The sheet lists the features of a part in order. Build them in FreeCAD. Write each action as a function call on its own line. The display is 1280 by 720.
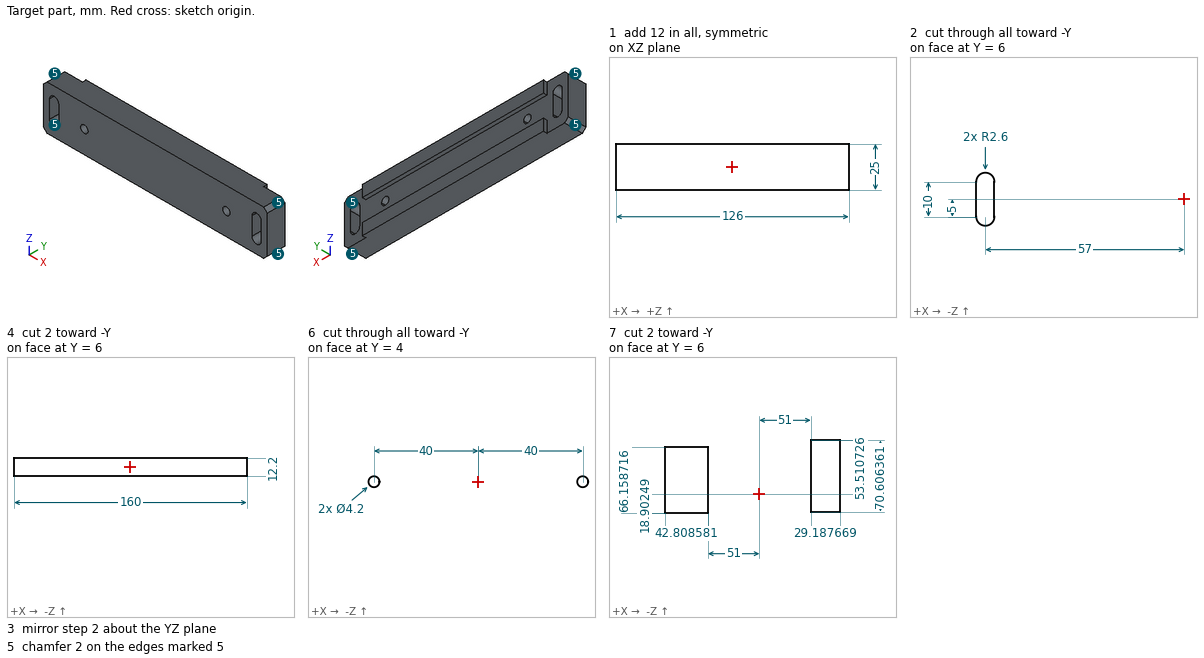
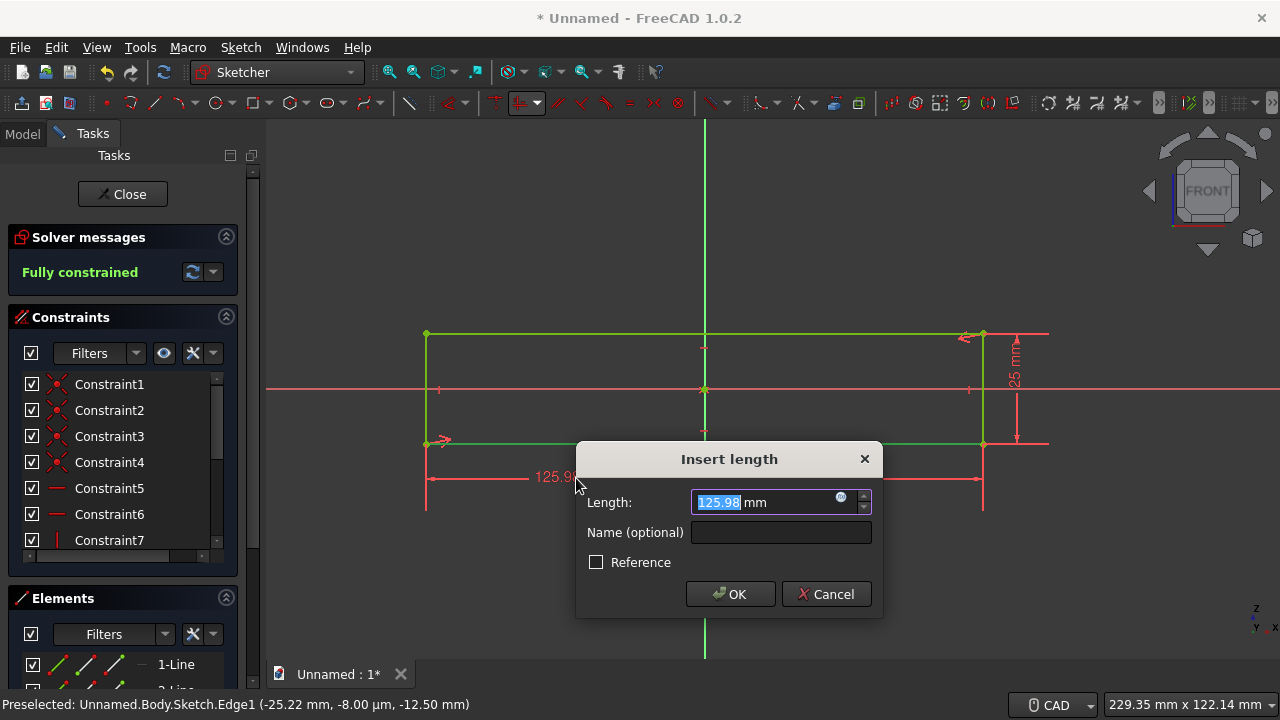
text(126)
key(Return)
key(Escape)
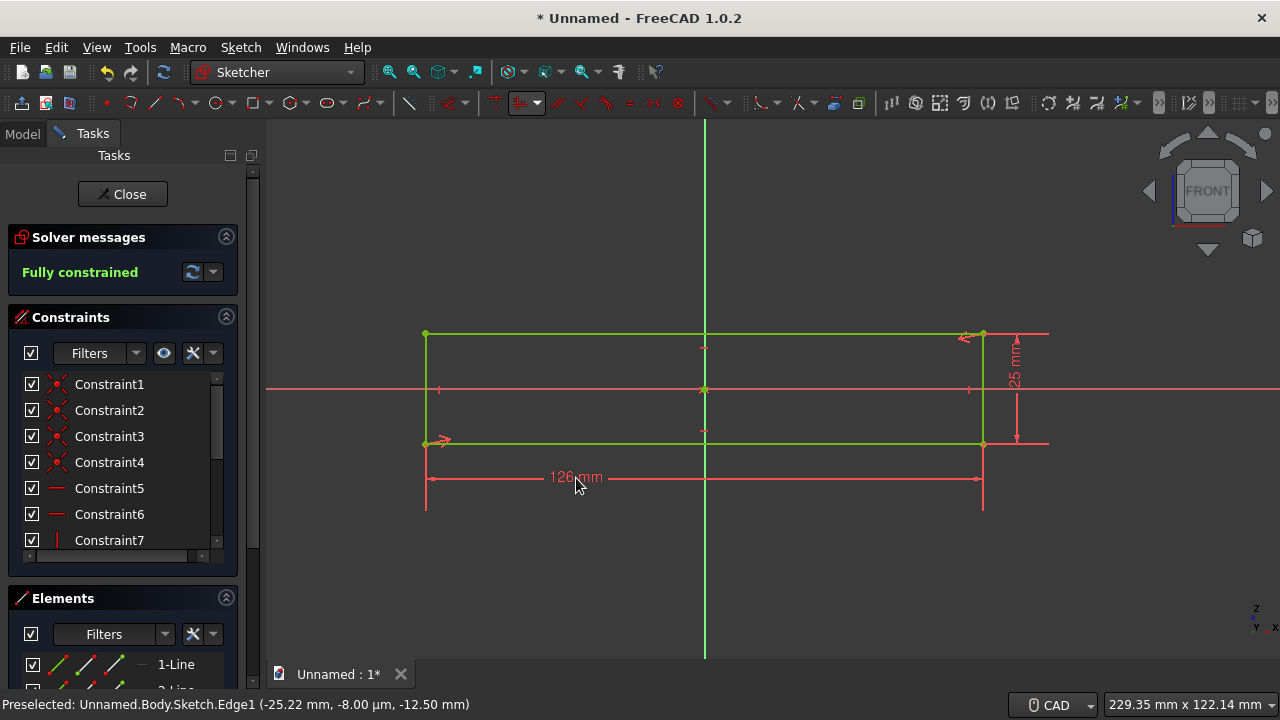
click(123, 194)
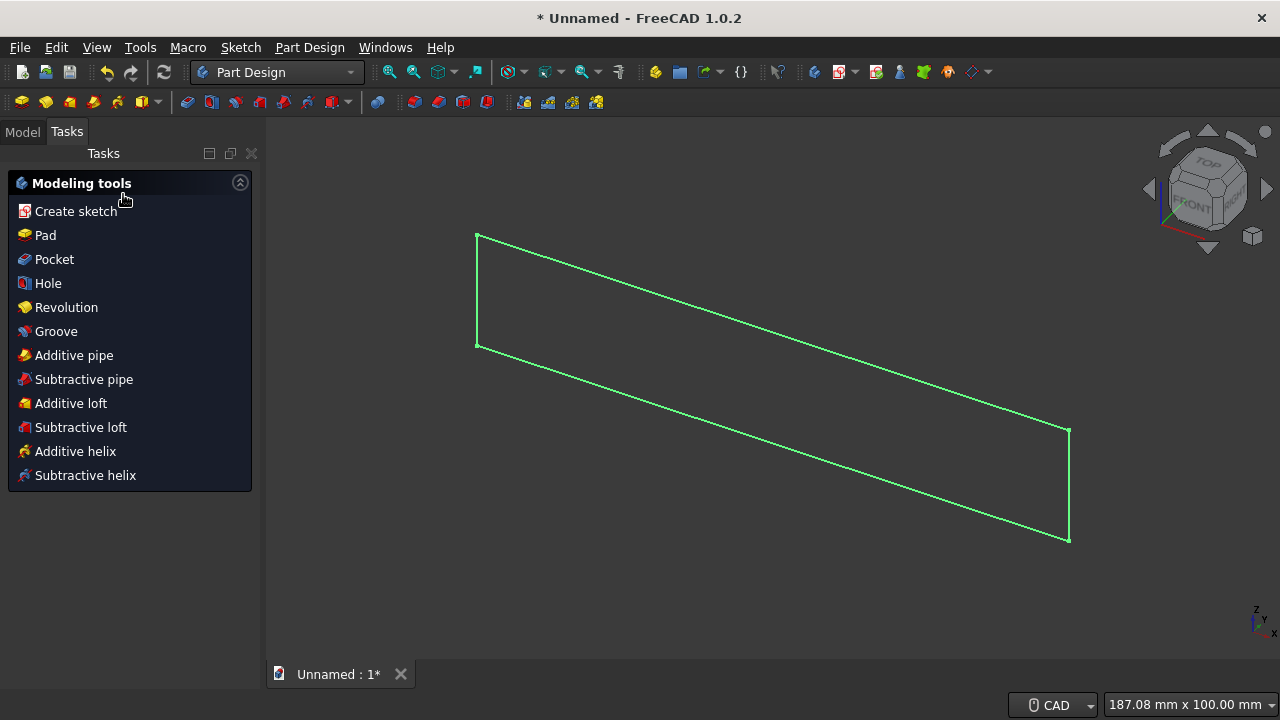
click(22, 102)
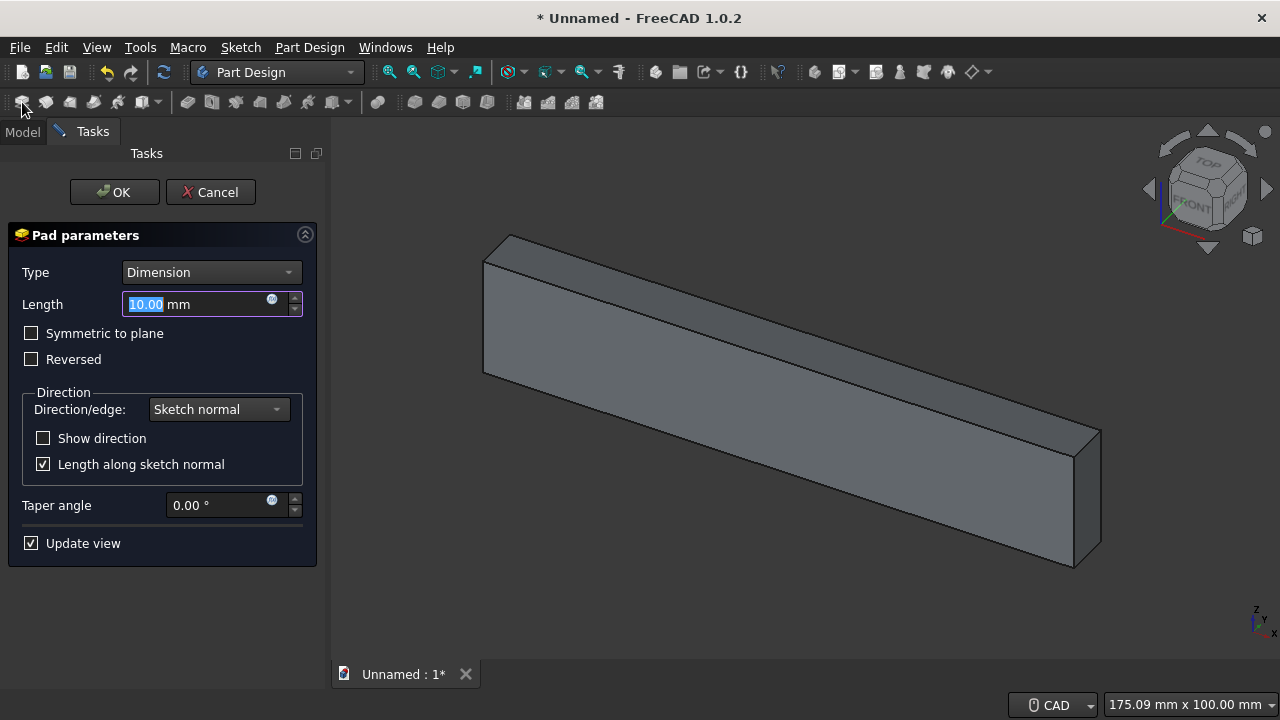
text(12)
key(Tab)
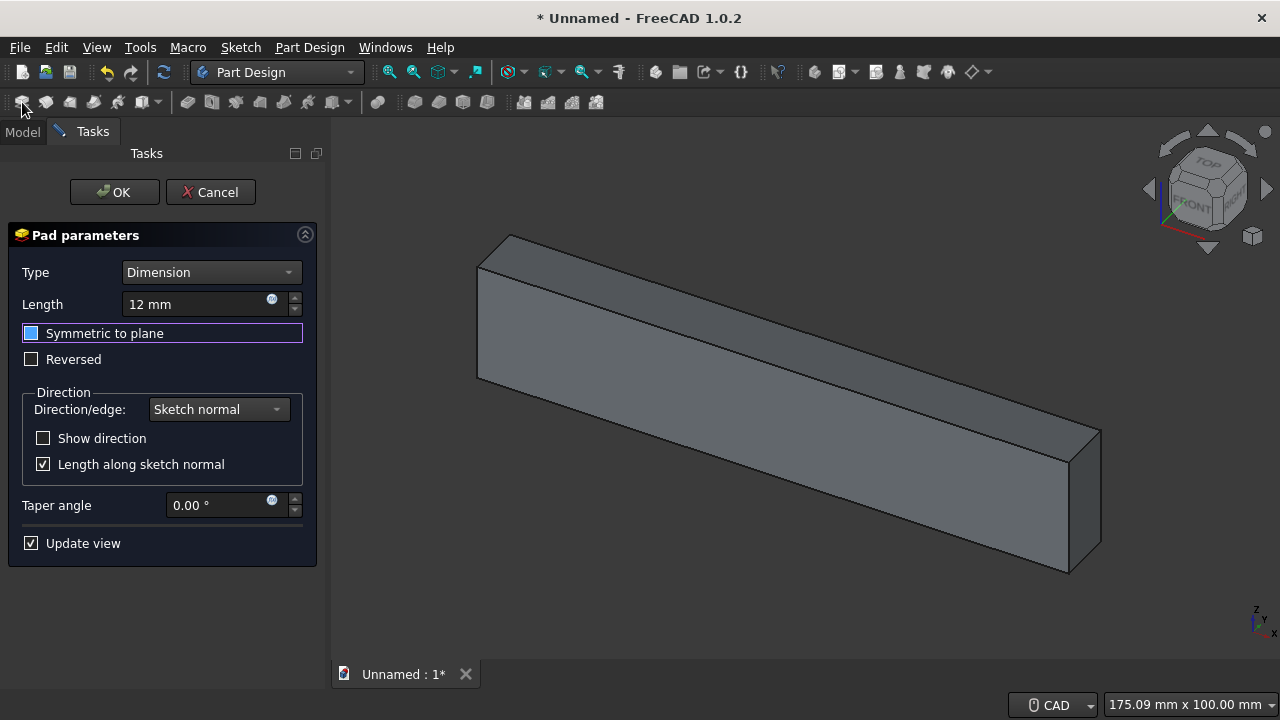
click(30, 333)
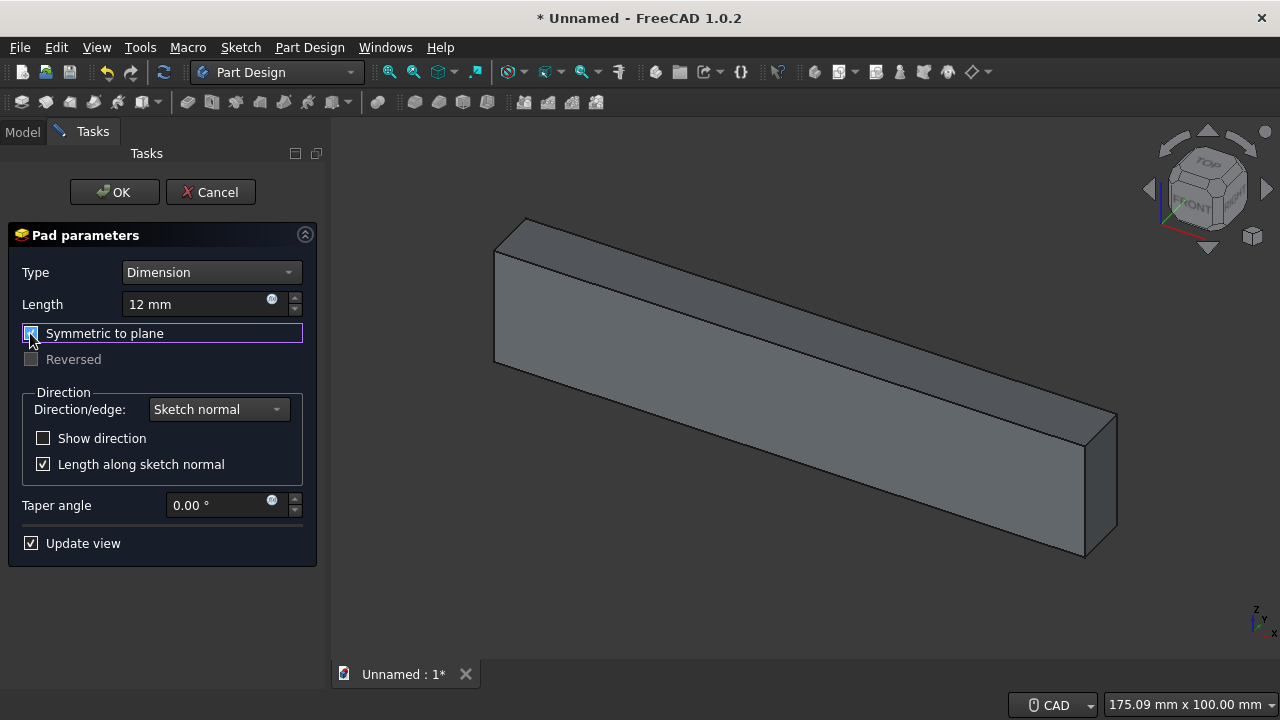
click(115, 192)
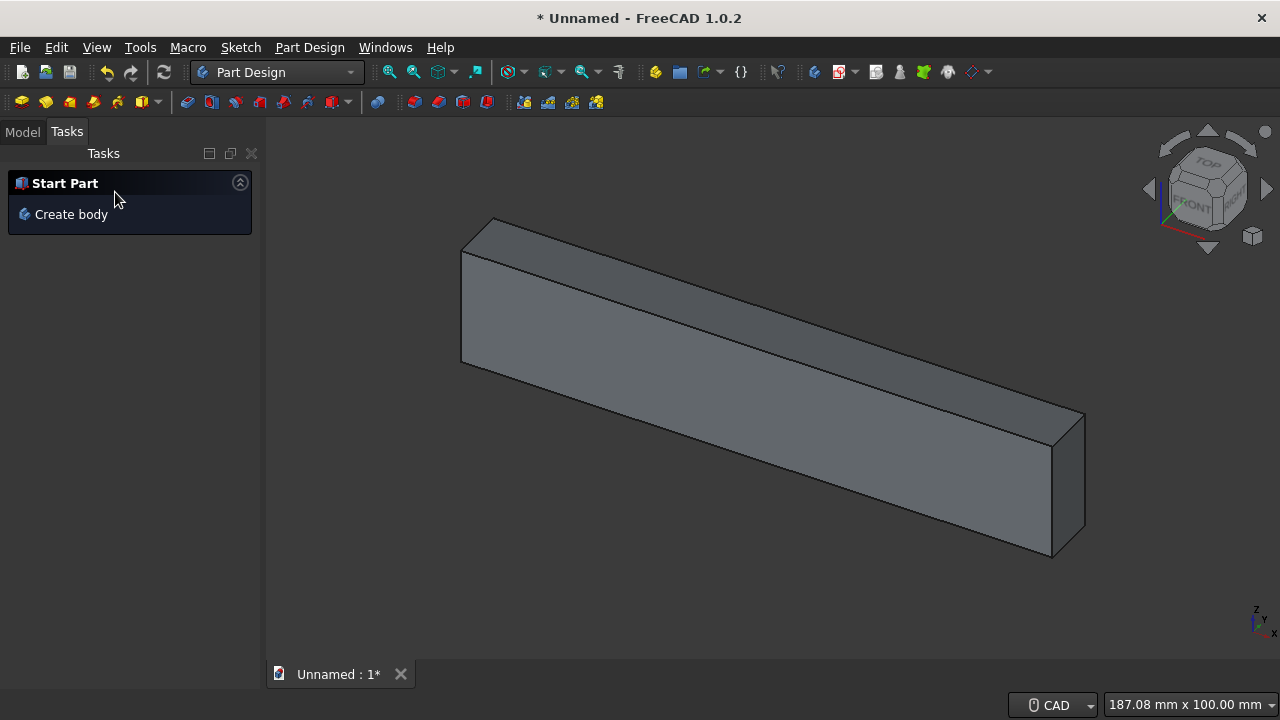
key(4)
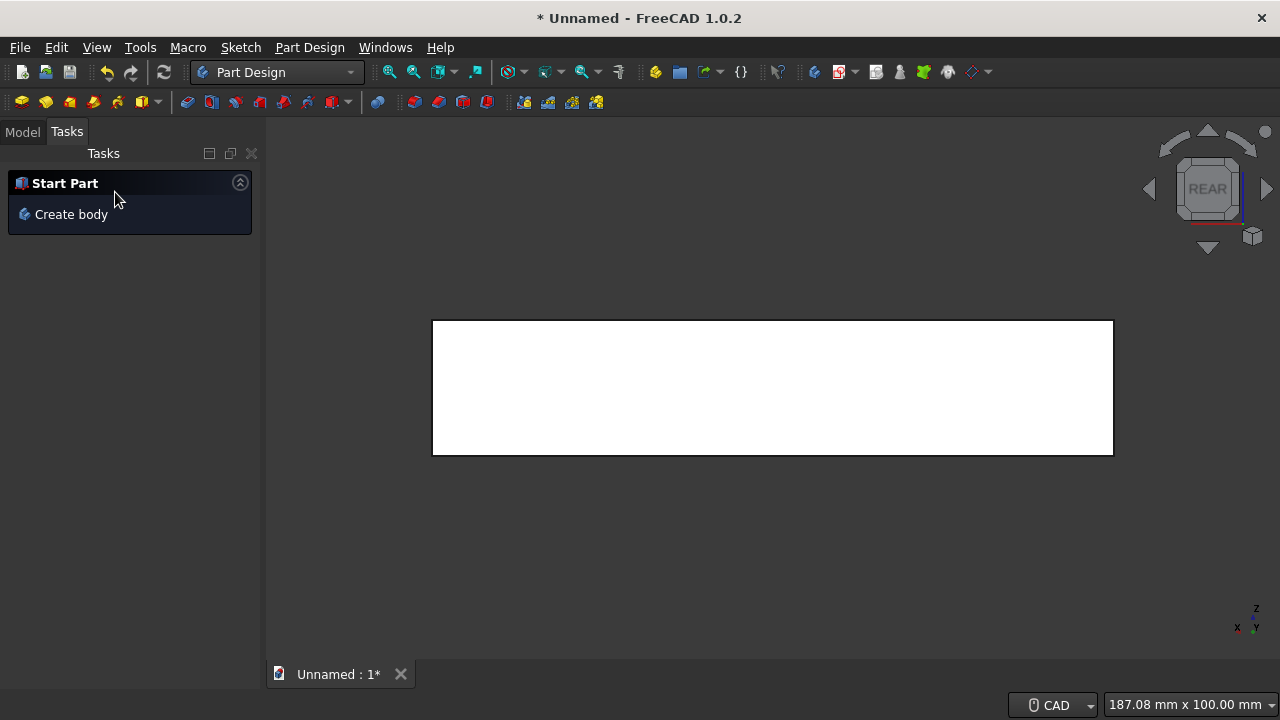
click(578, 387)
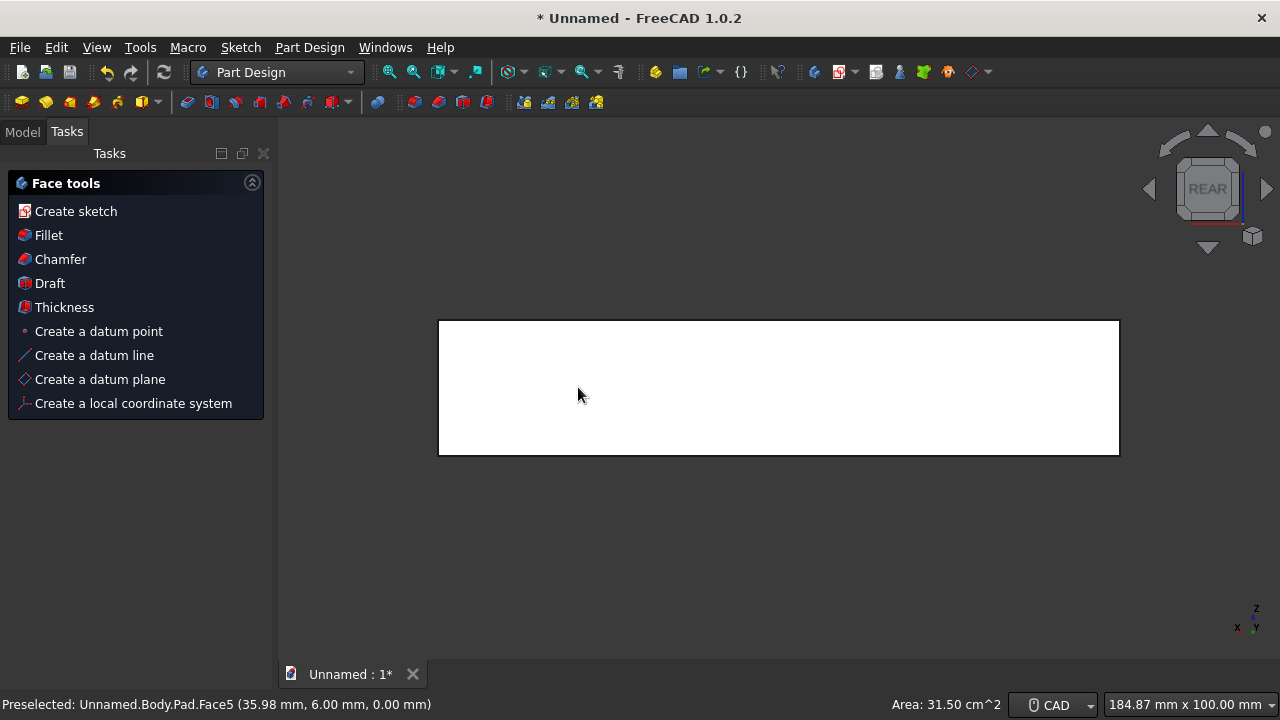
click(840, 72)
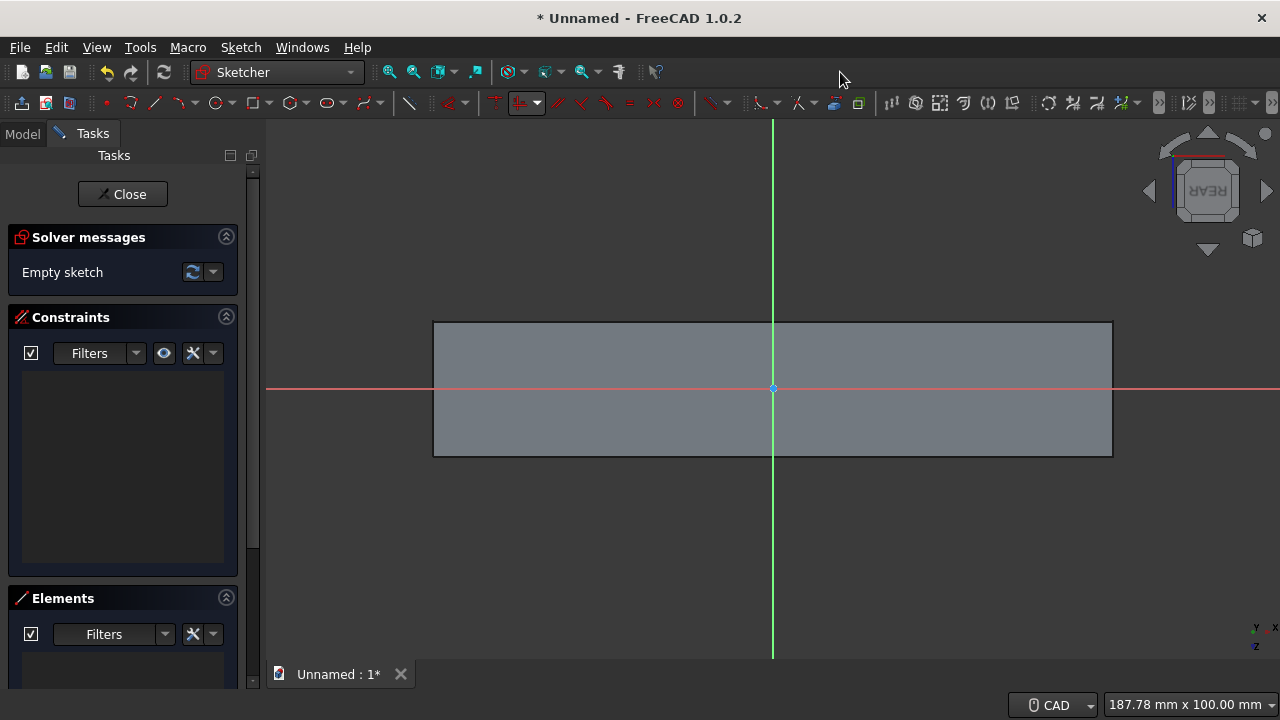
scroll(387, 389, up, 7)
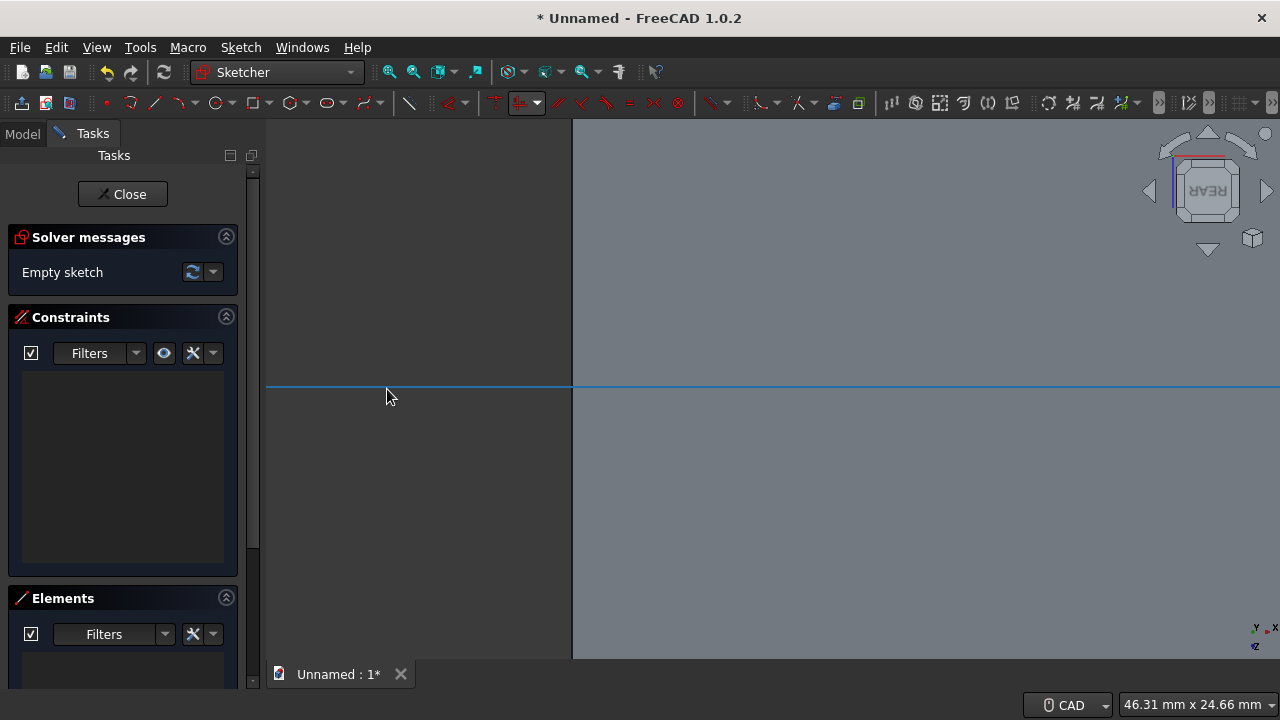
click(328, 104)